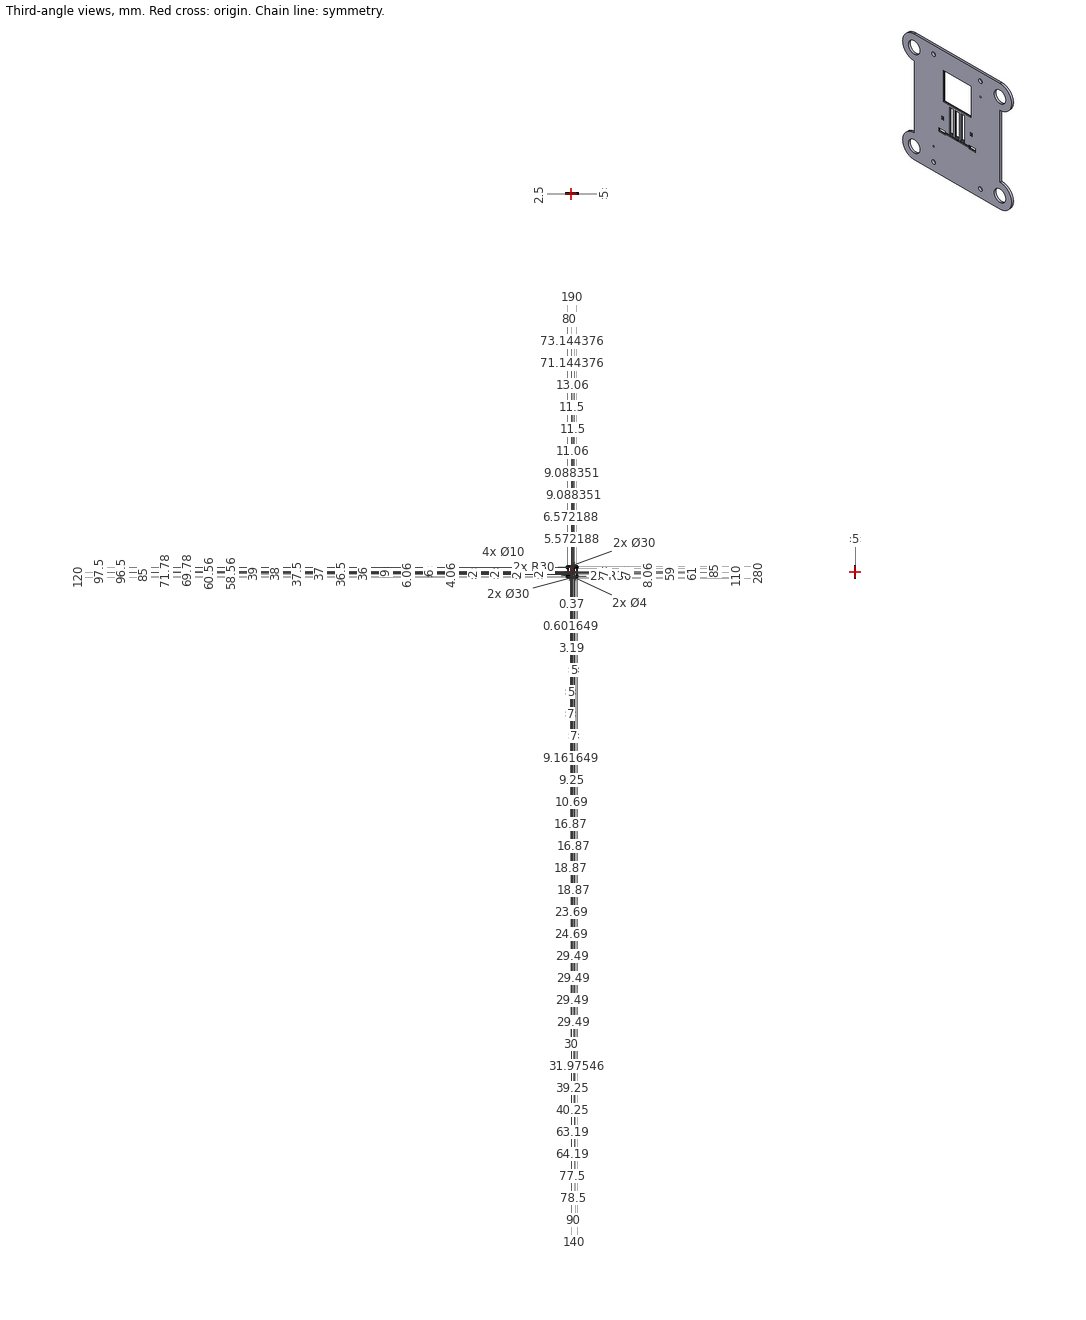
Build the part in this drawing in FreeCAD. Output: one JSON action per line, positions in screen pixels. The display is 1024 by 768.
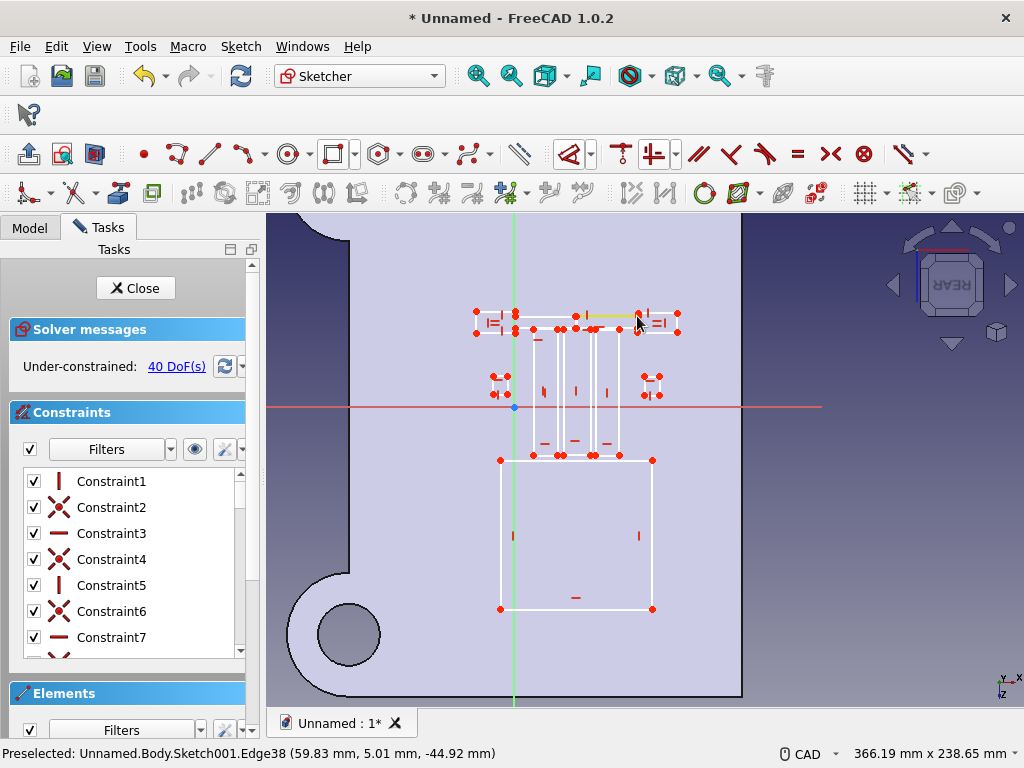
{"action": "scroll", "coordinate": [515, 332], "scroll_direction": "up", "scroll_amount": 14}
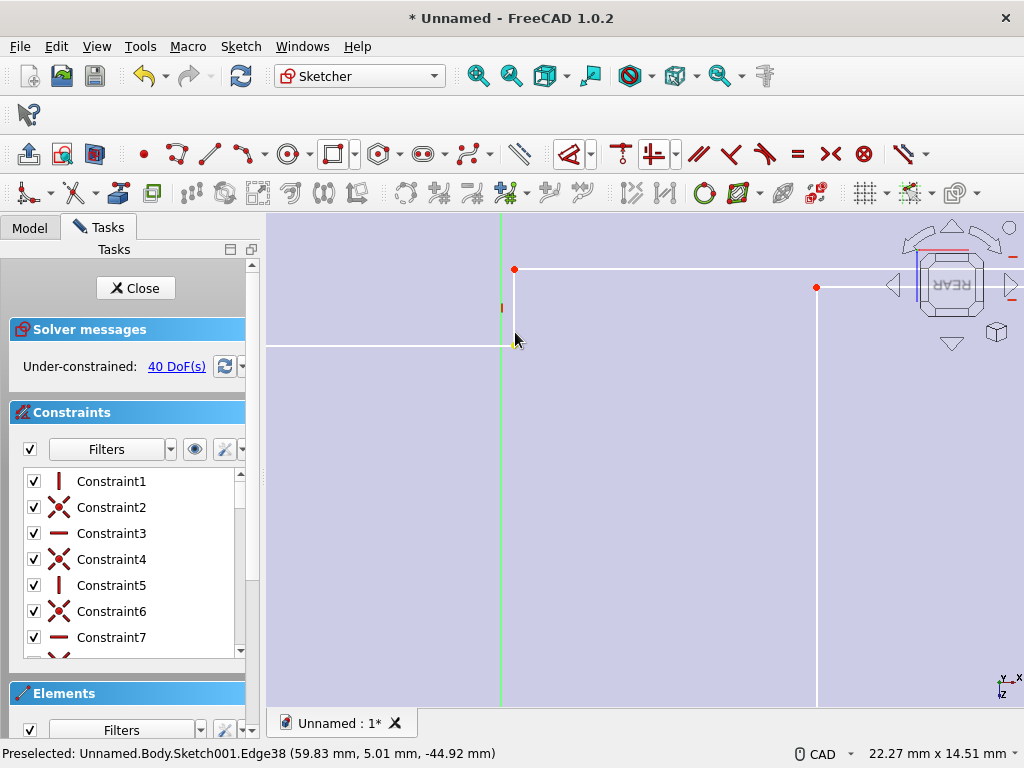
{"action": "left_click", "coordinate": [514, 323]}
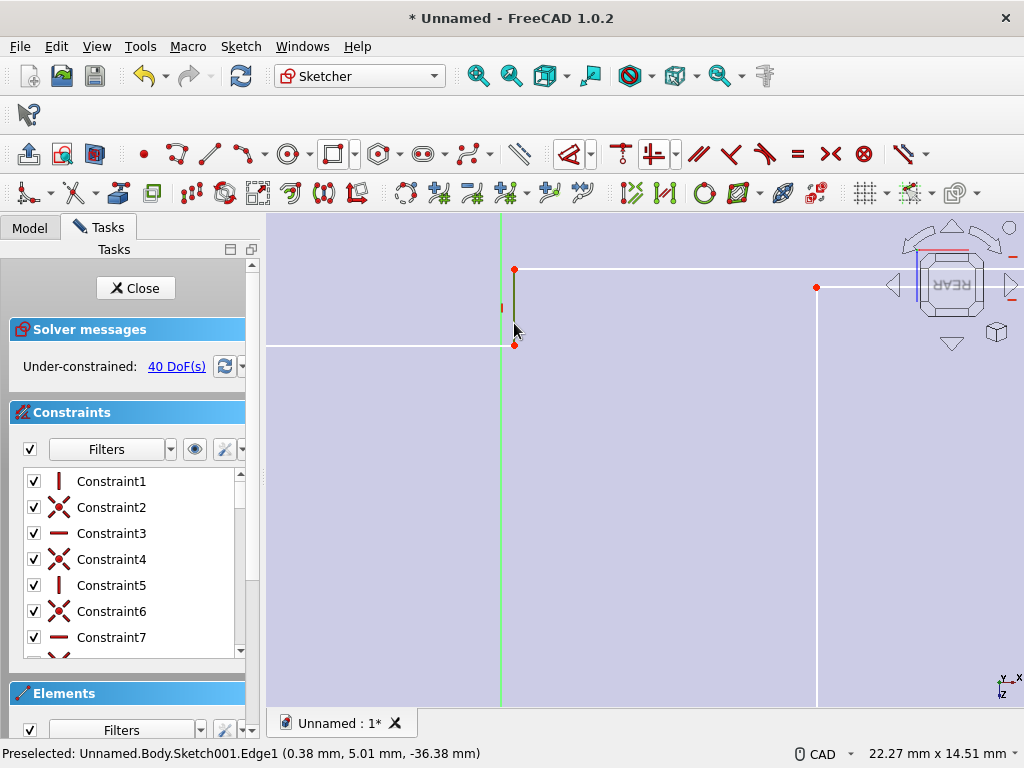
{"action": "left_click", "coordinate": [590, 154]}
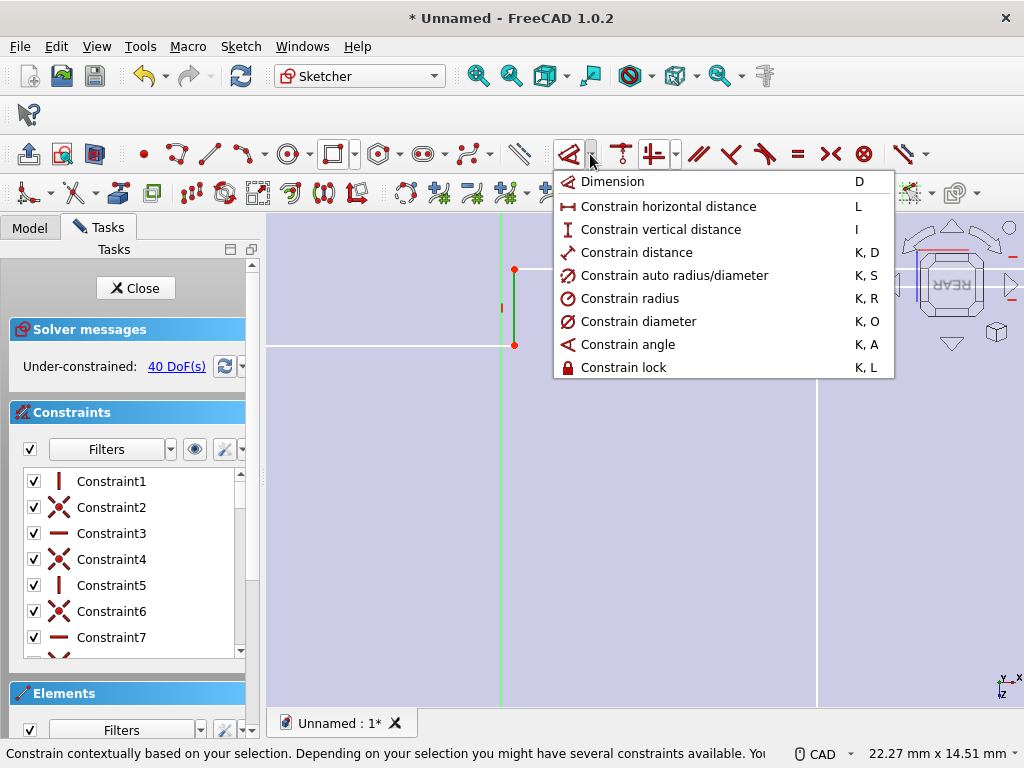
{"action": "left_click", "coordinate": [724, 230]}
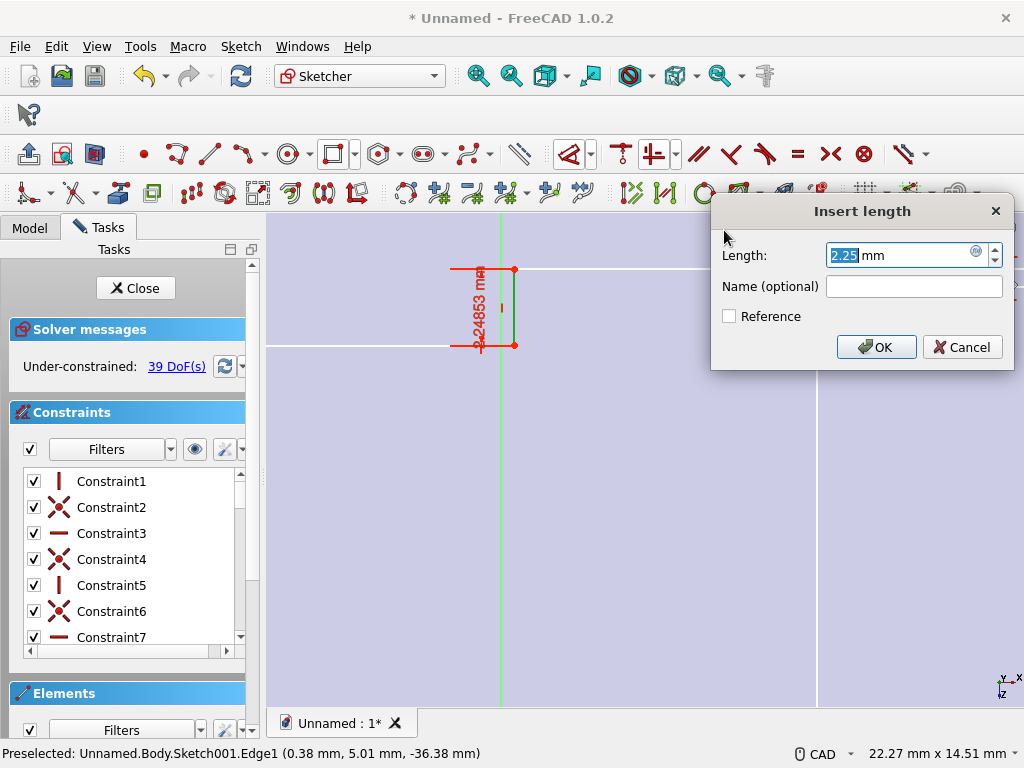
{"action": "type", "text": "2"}
{"action": "key", "text": "Return"}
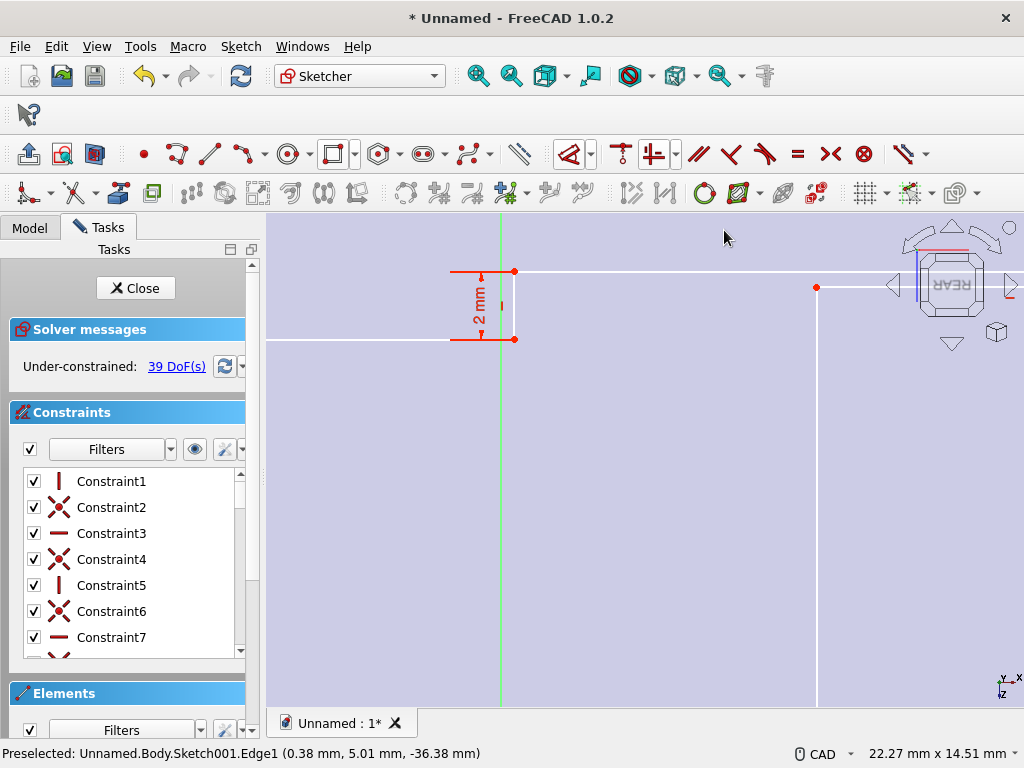
{"action": "scroll", "coordinate": [515, 332], "scroll_direction": "down", "scroll_amount": 14}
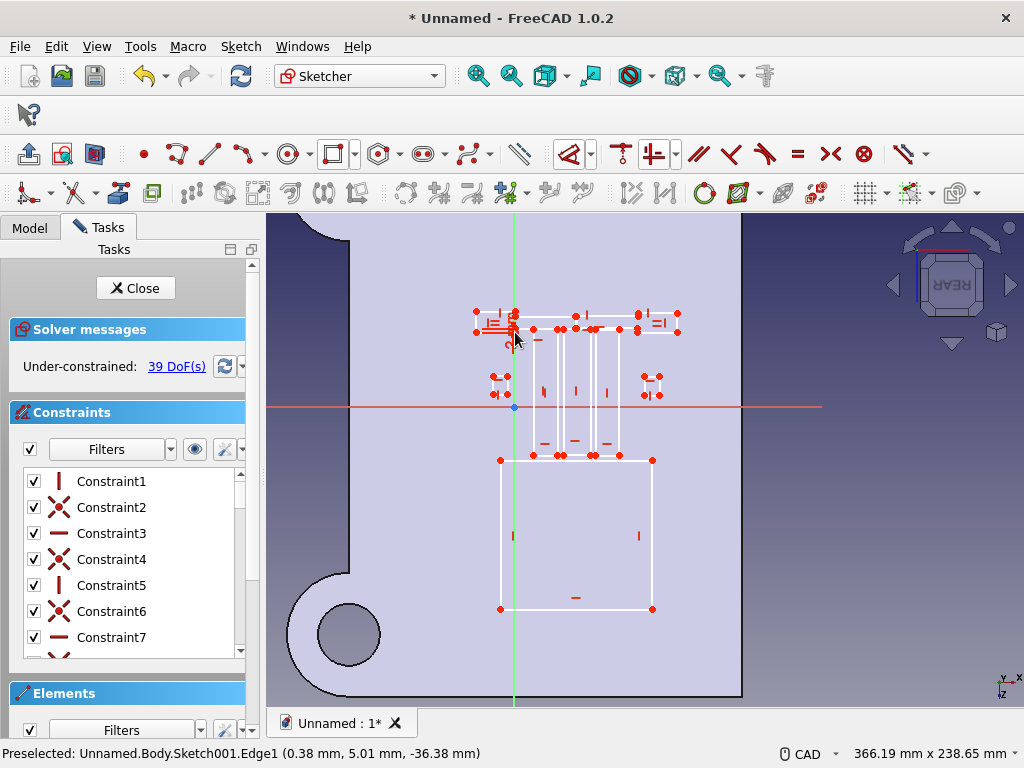
{"action": "scroll", "coordinate": [515, 315], "scroll_direction": "up", "scroll_amount": 14}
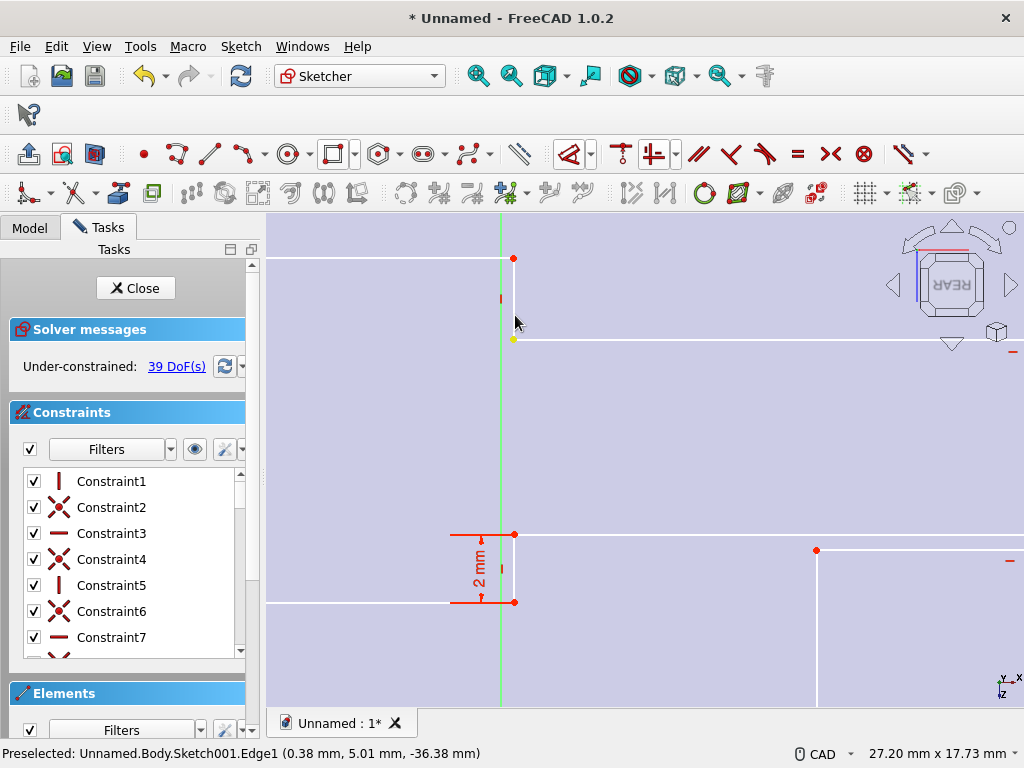
{"action": "left_click", "coordinate": [514, 315]}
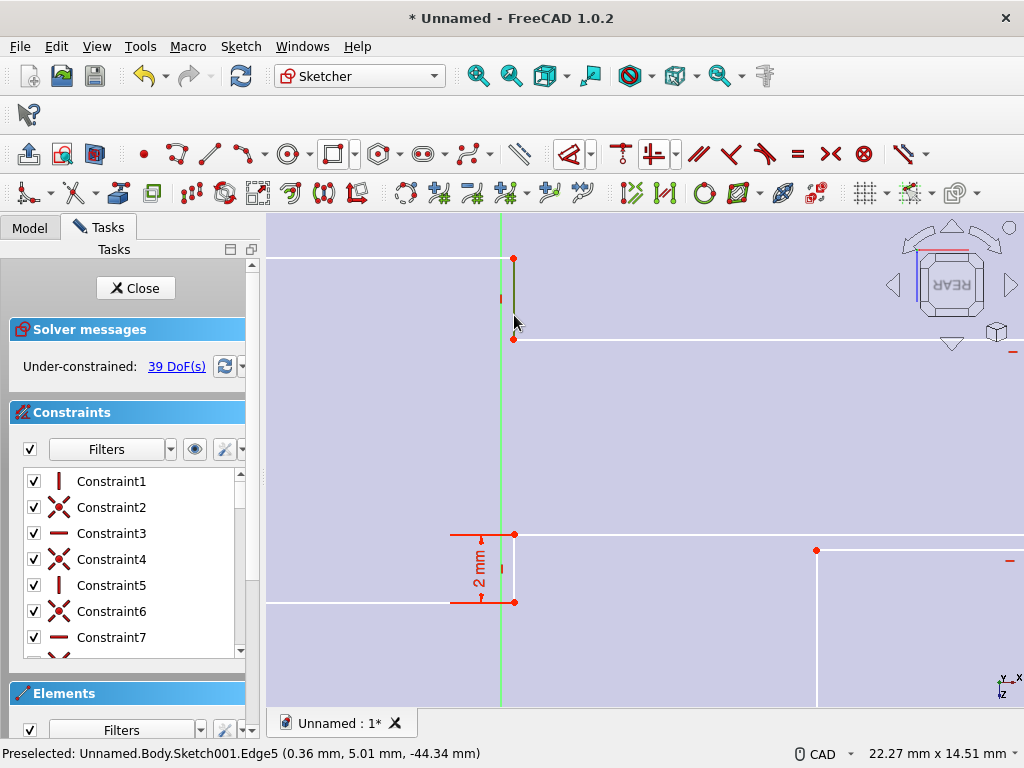
{"action": "left_click", "coordinate": [590, 154]}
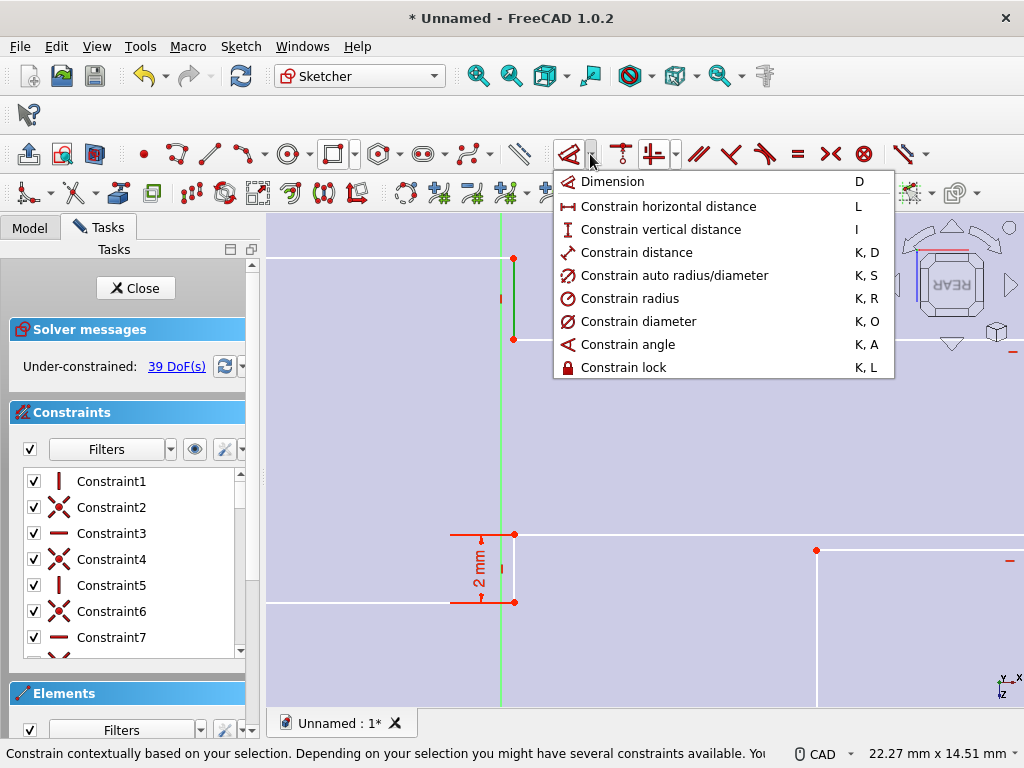
{"action": "left_click", "coordinate": [724, 230]}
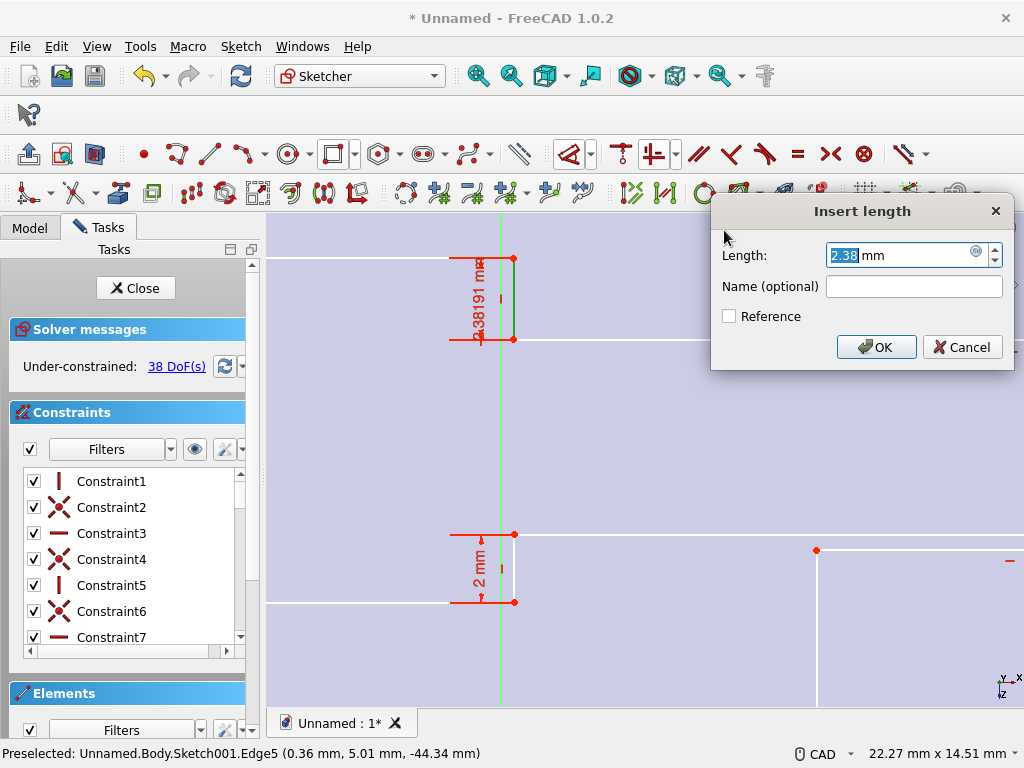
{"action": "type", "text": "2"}
{"action": "key", "text": "Return"}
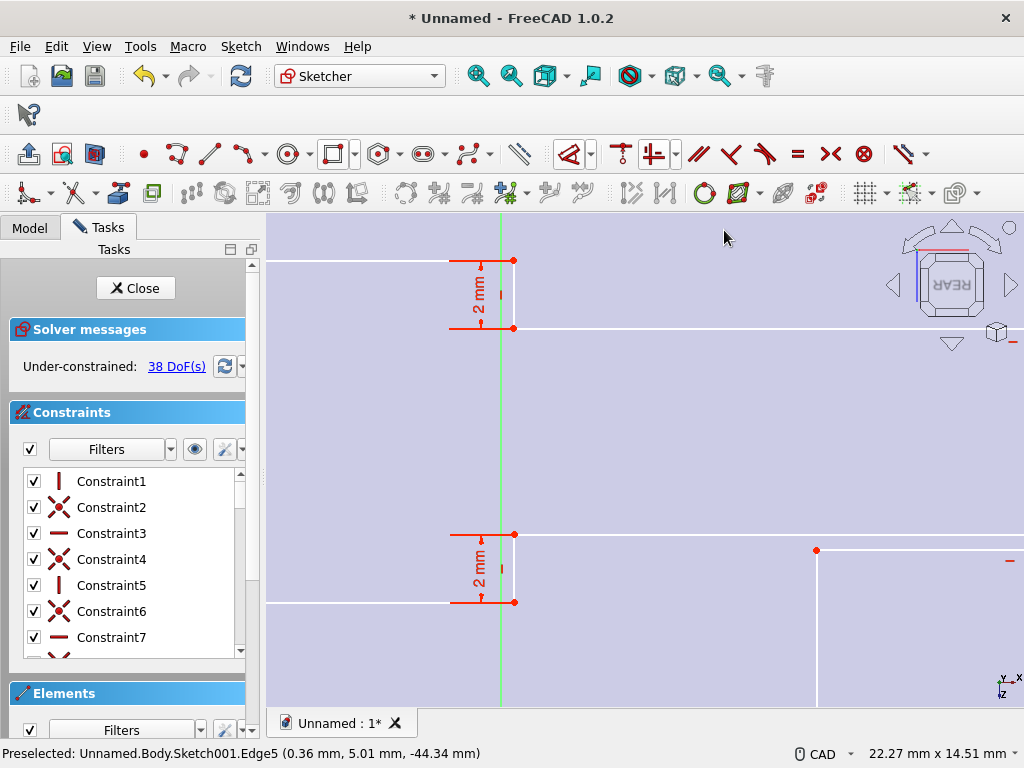
{"action": "scroll", "coordinate": [515, 315], "scroll_direction": "down", "scroll_amount": 14}